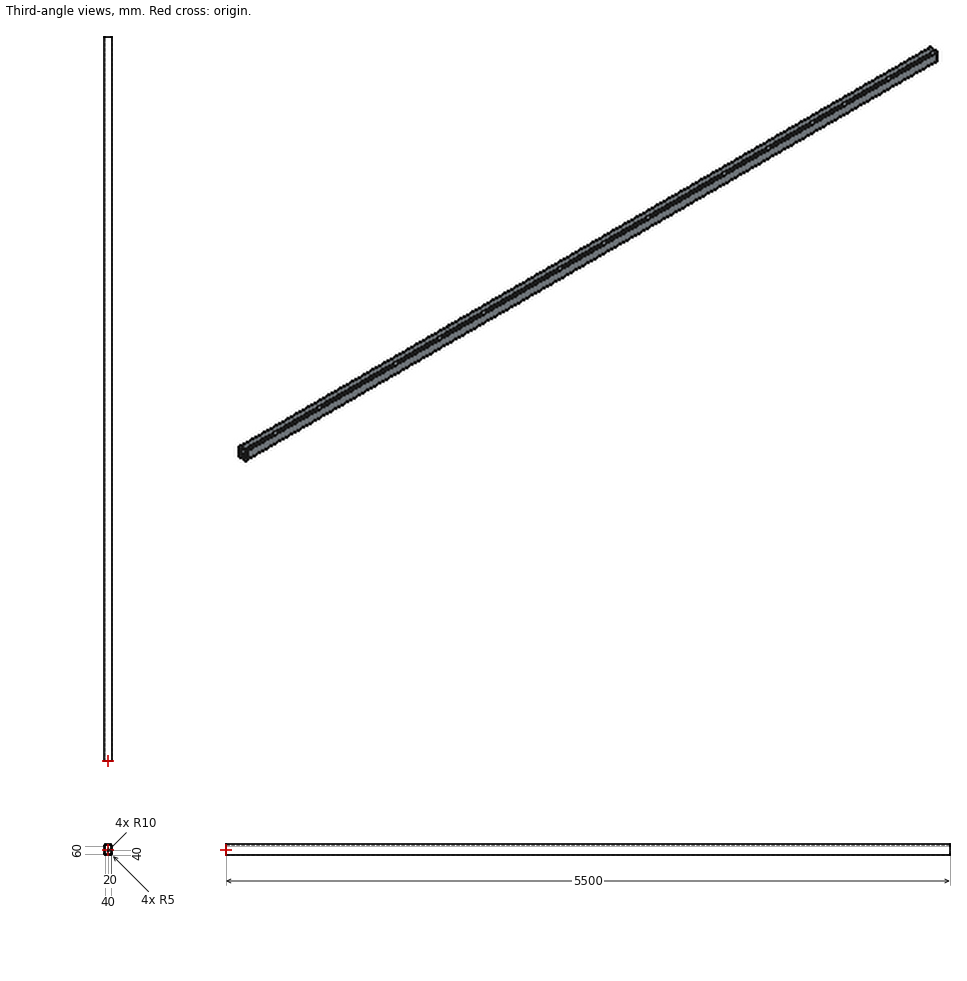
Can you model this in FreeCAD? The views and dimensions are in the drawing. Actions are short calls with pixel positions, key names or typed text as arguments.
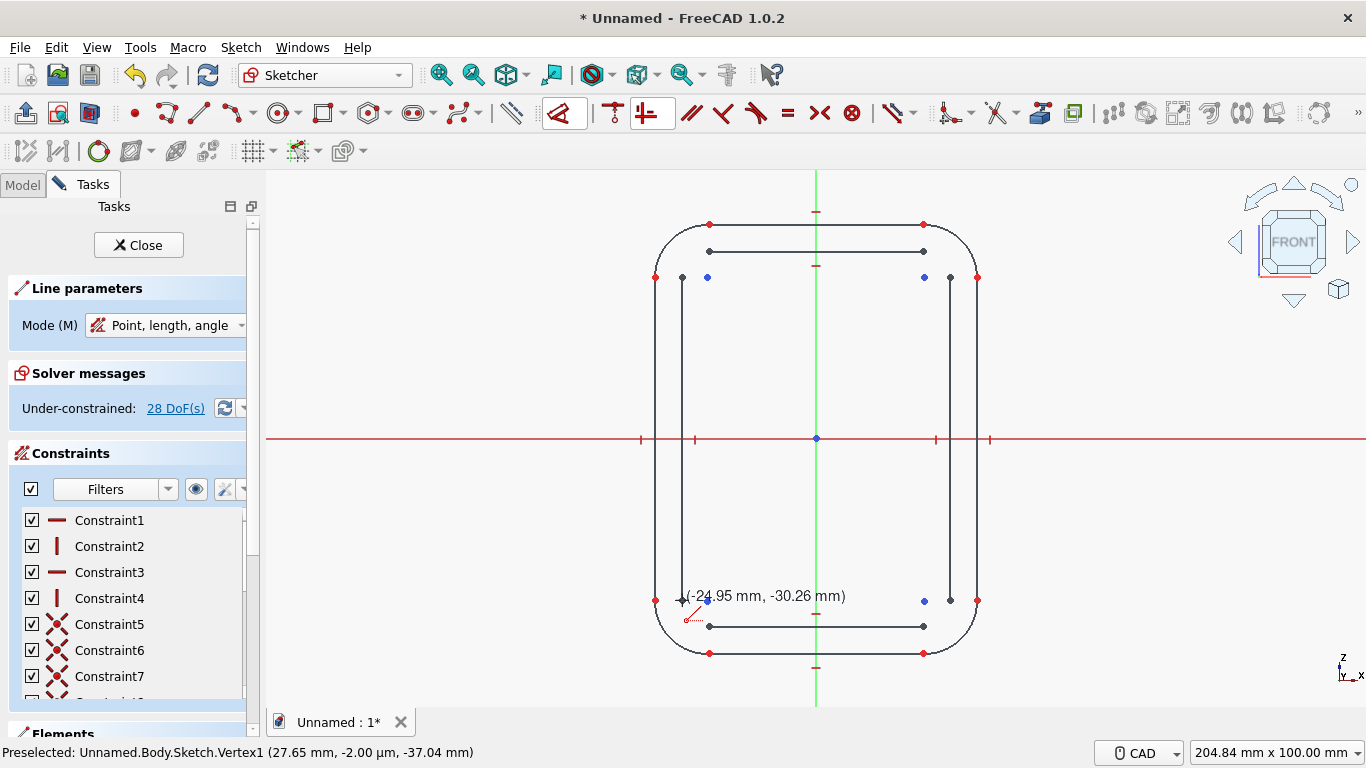
click(232, 114)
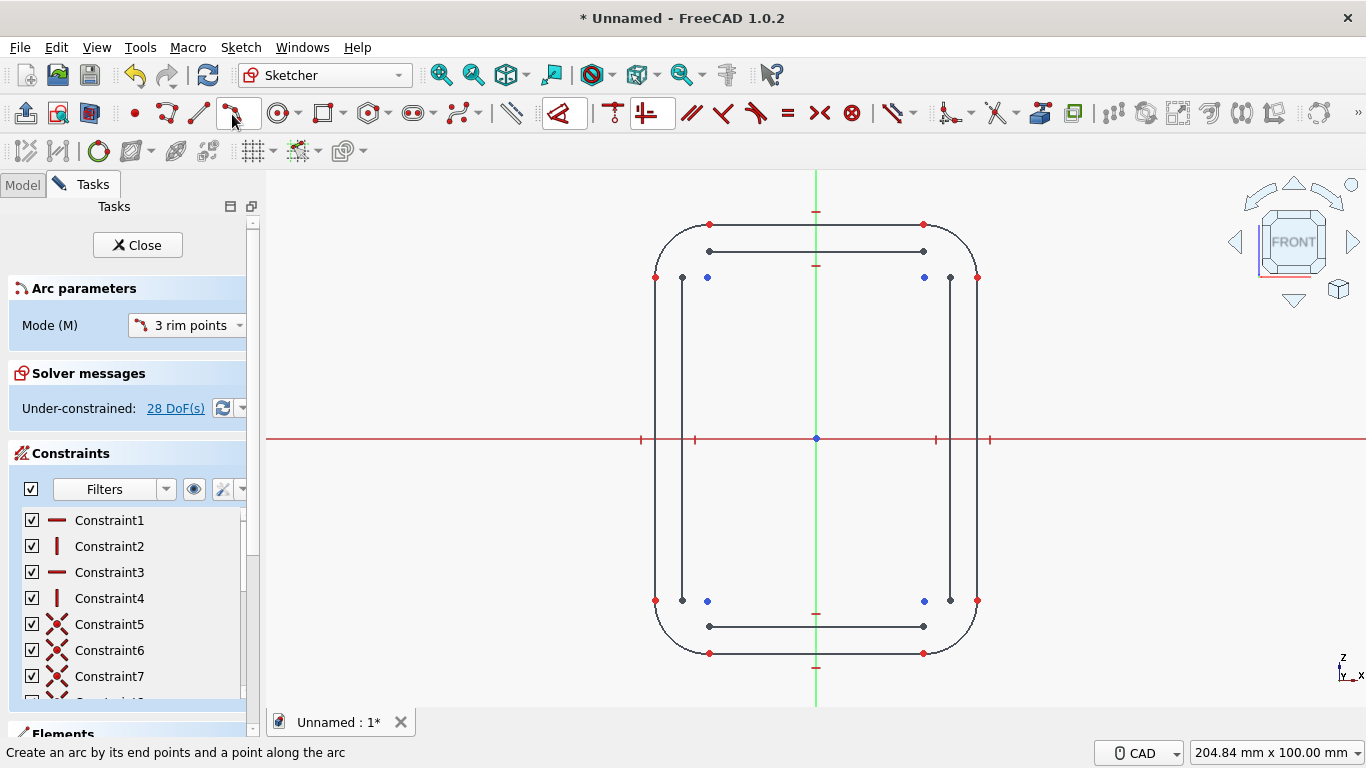
click(923, 627)
click(950, 601)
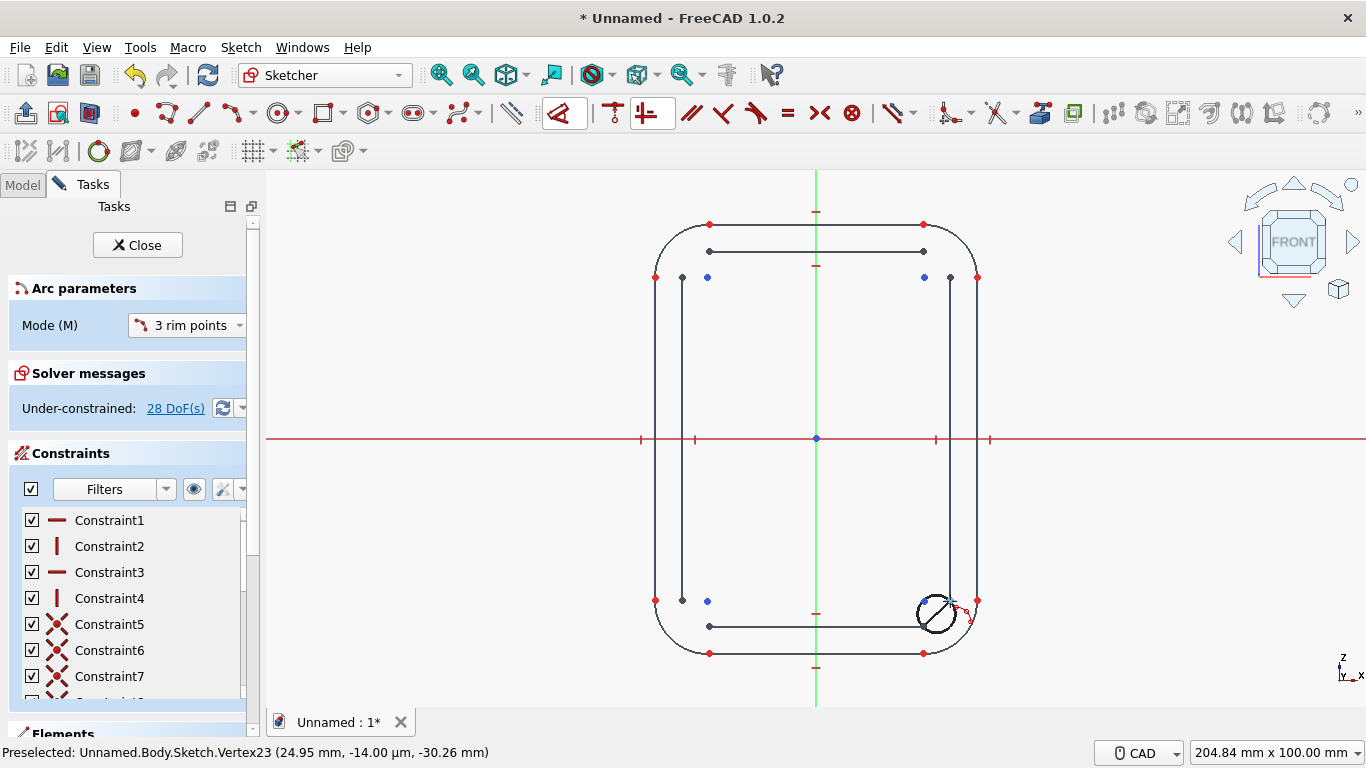
scroll(942, 619, up, 4)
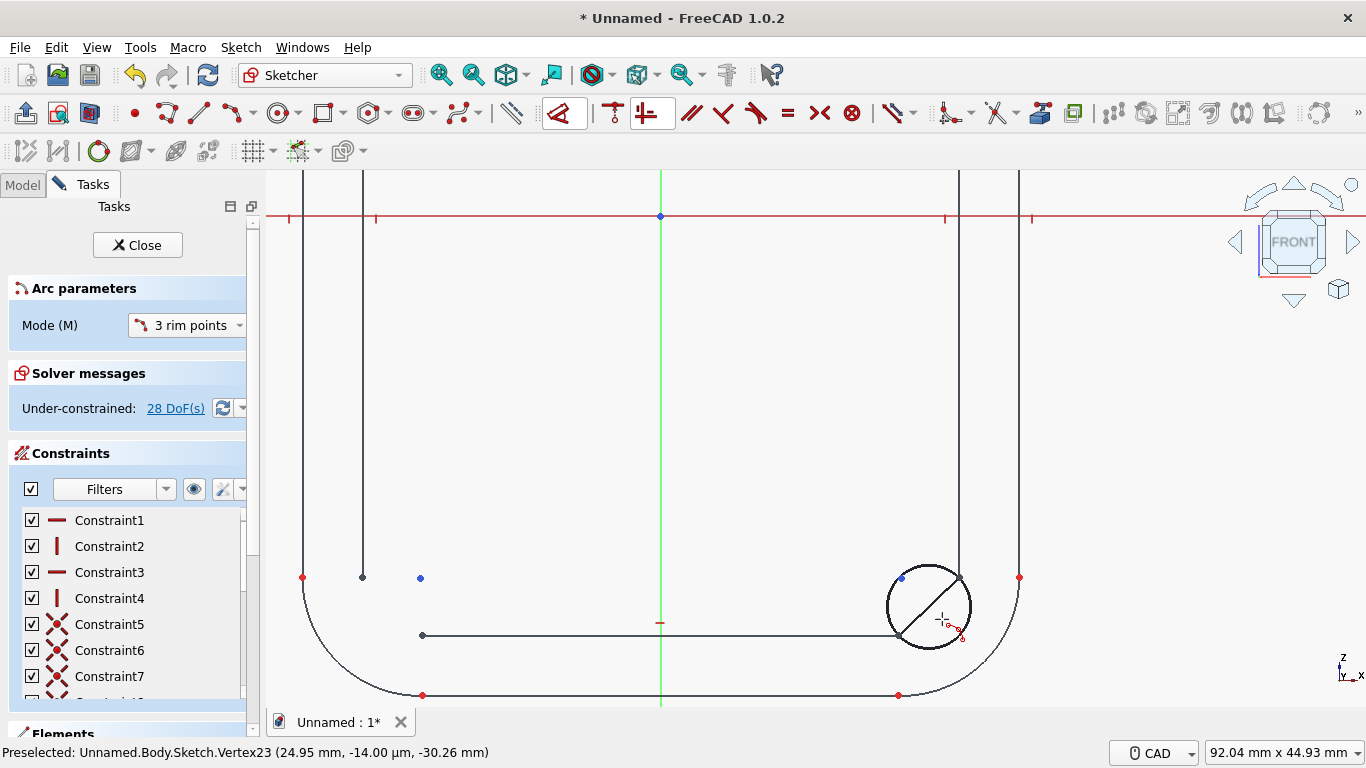
click(942, 617)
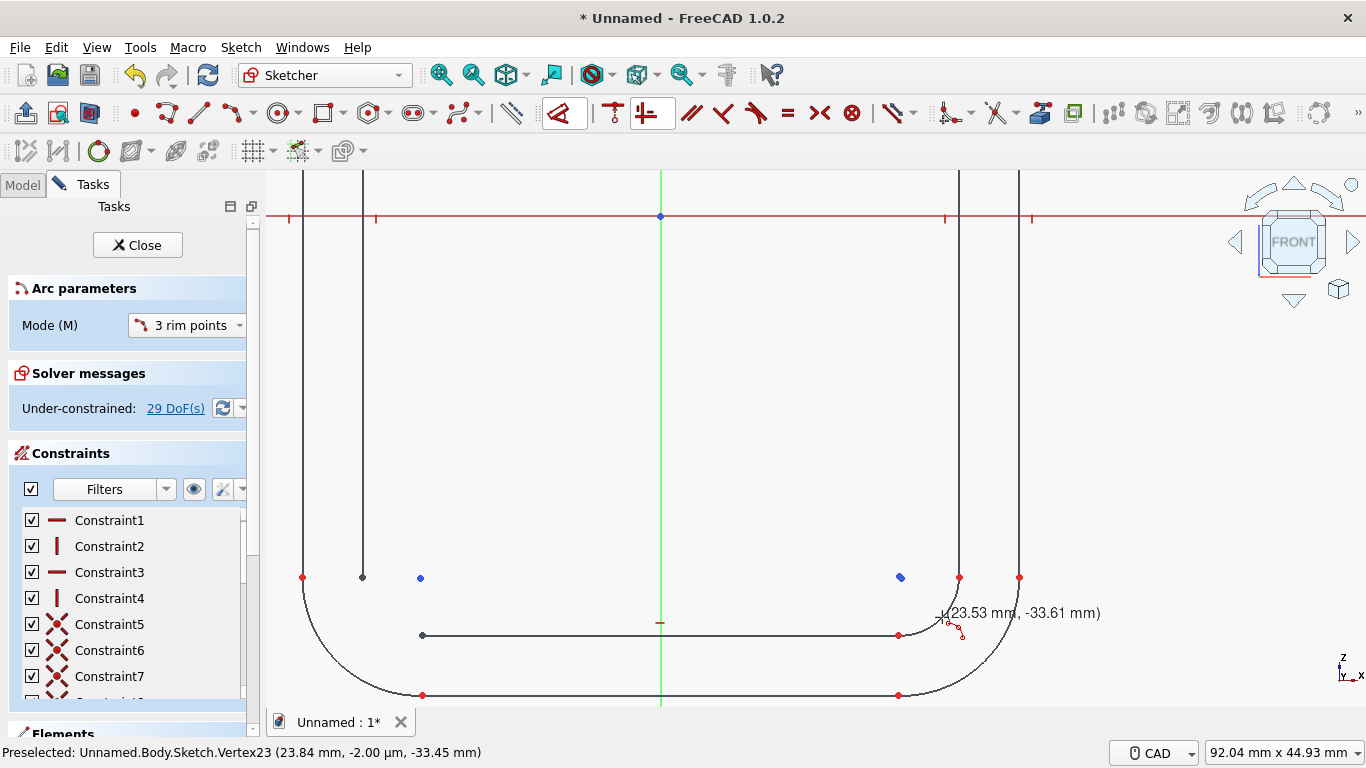
scroll(798, 568, down, 5)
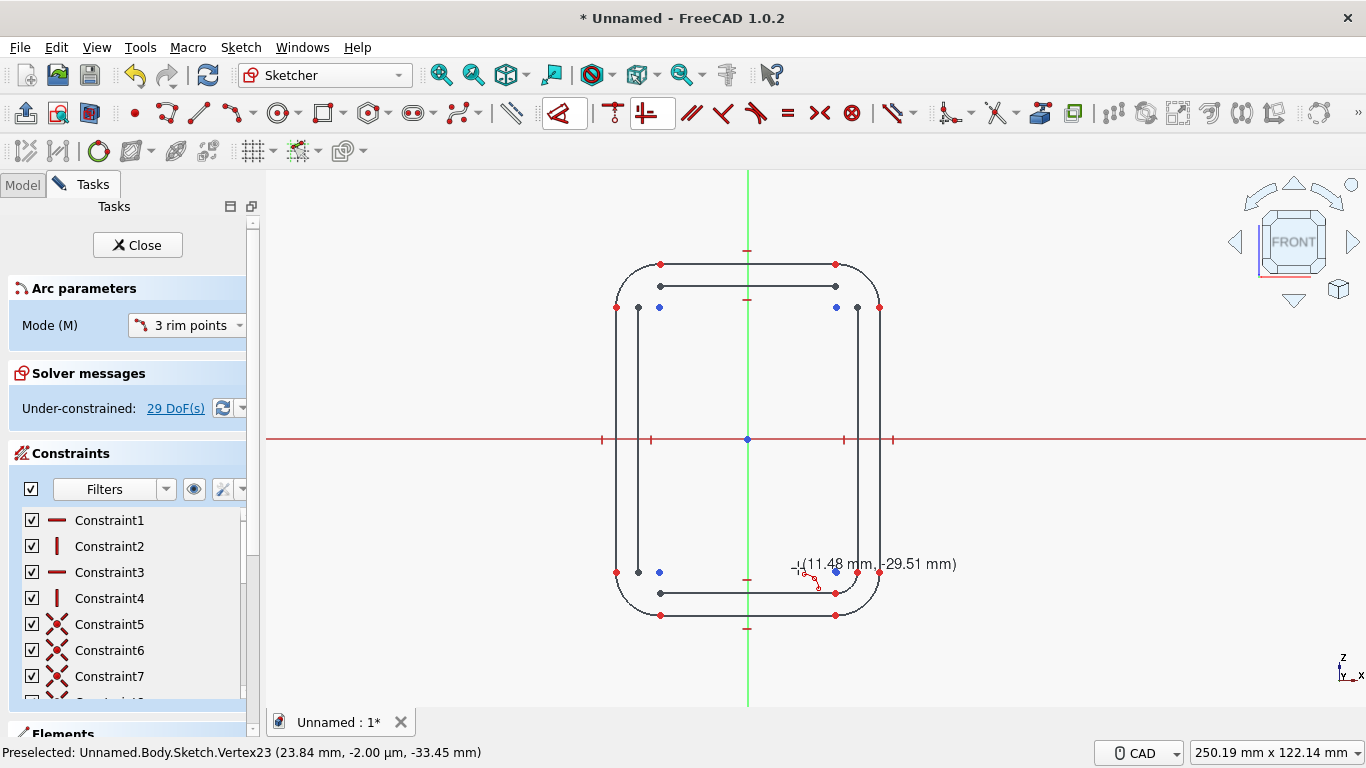
click(858, 308)
click(835, 286)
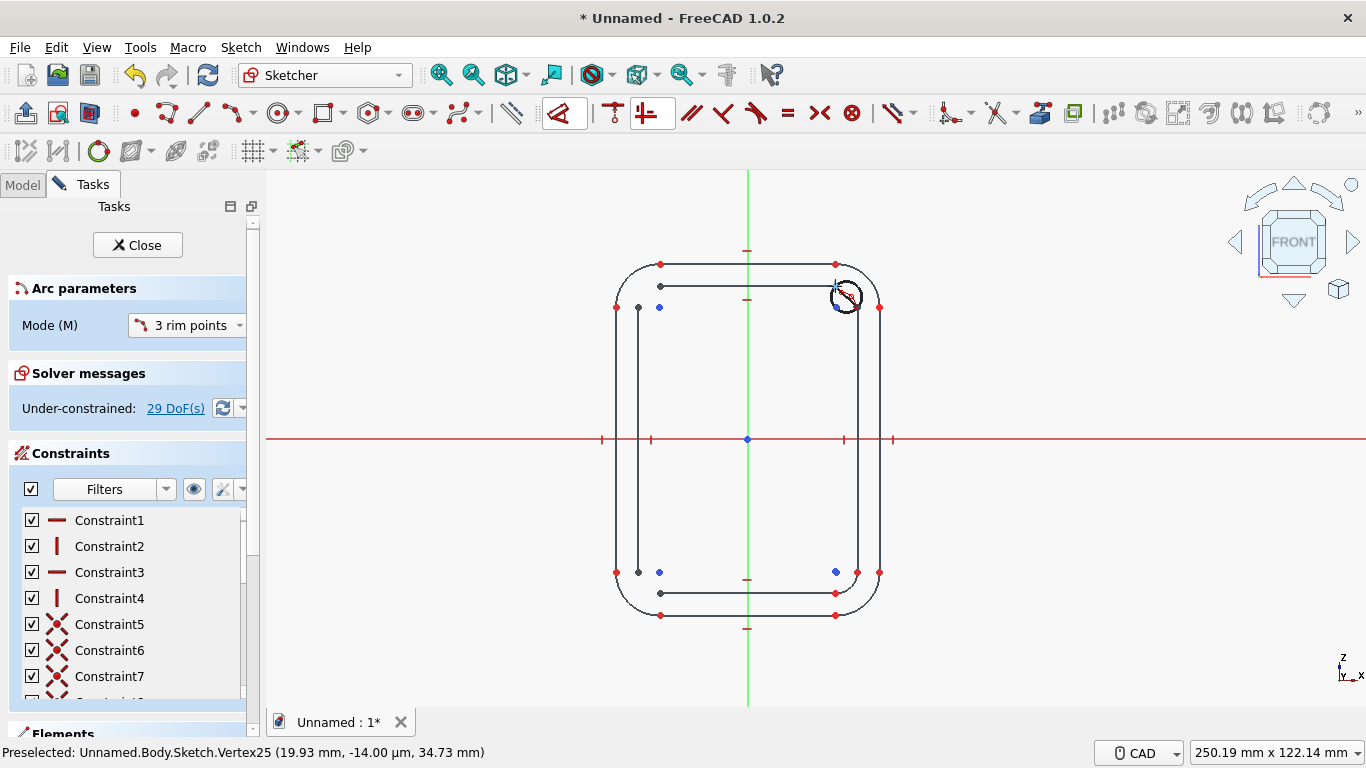
scroll(851, 292, up, 5)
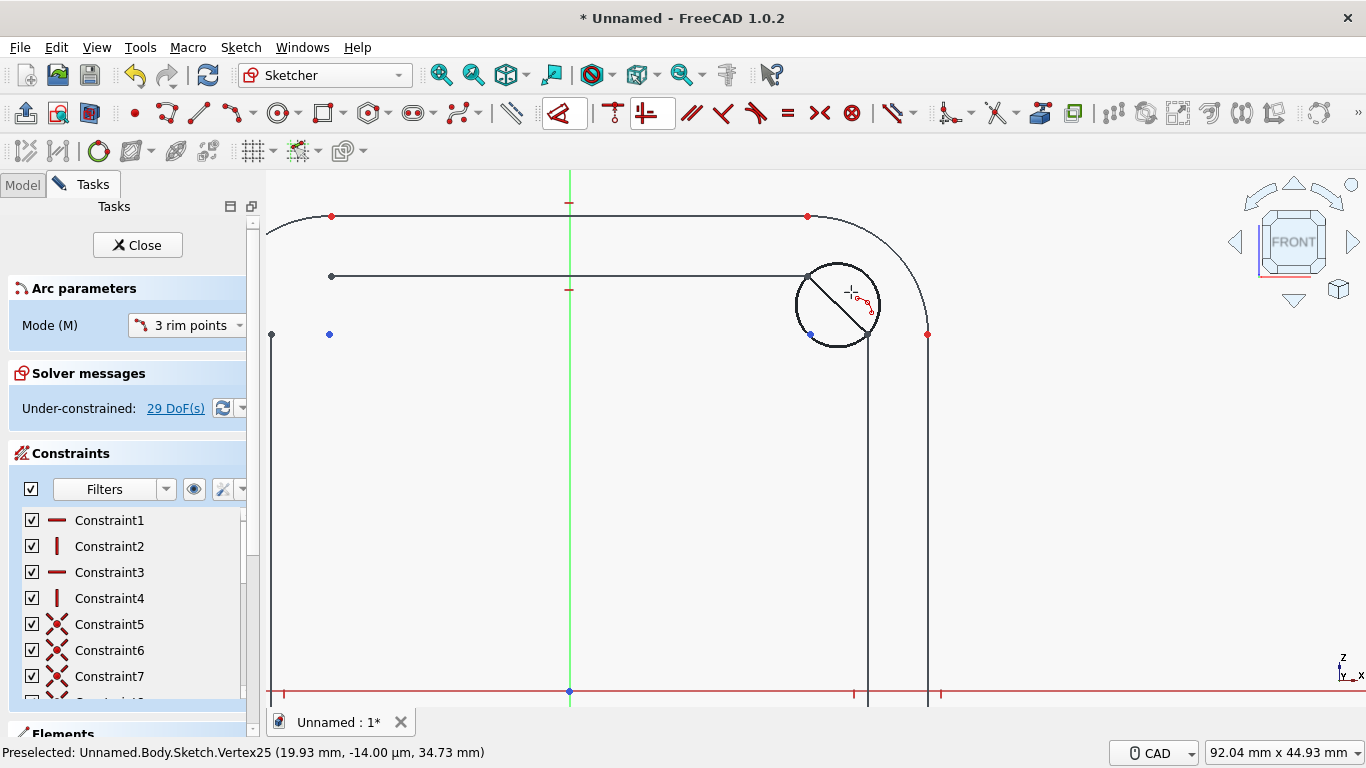
click(851, 291)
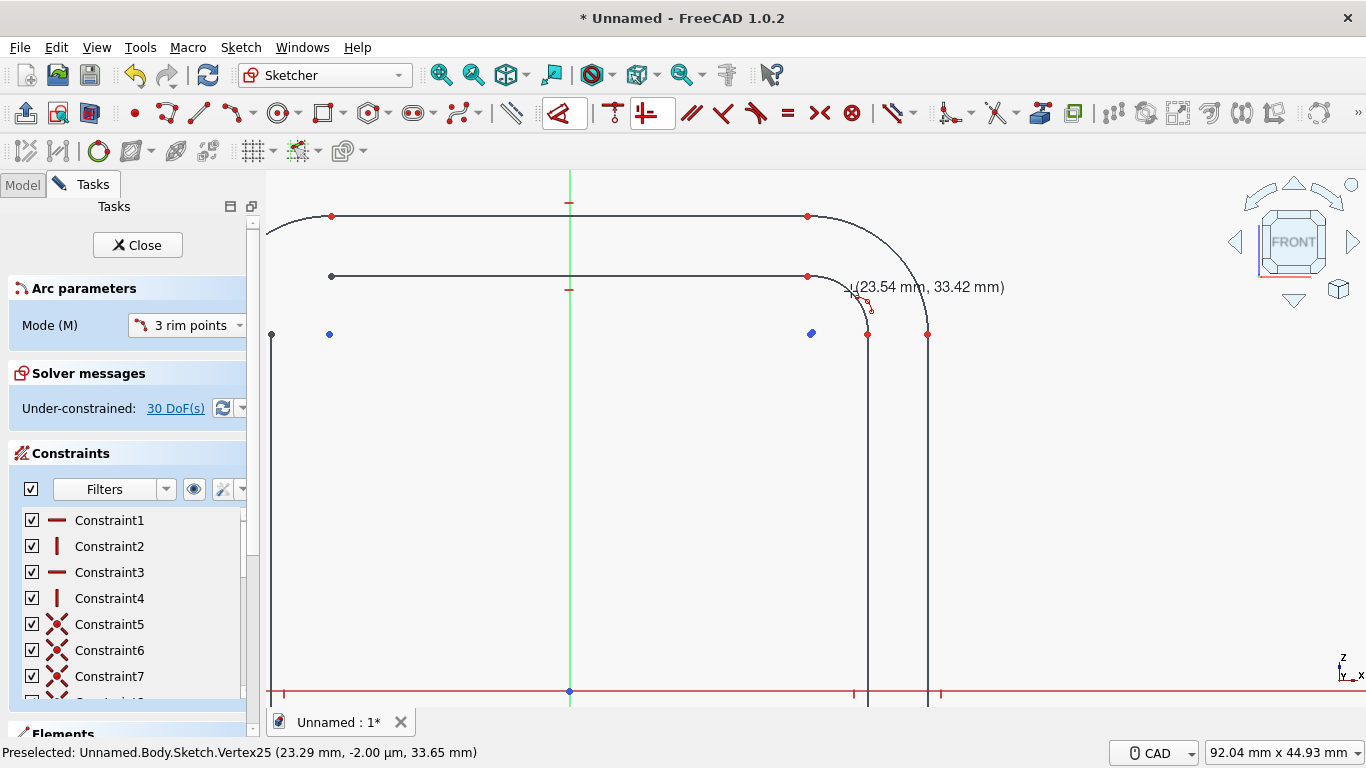
click(332, 276)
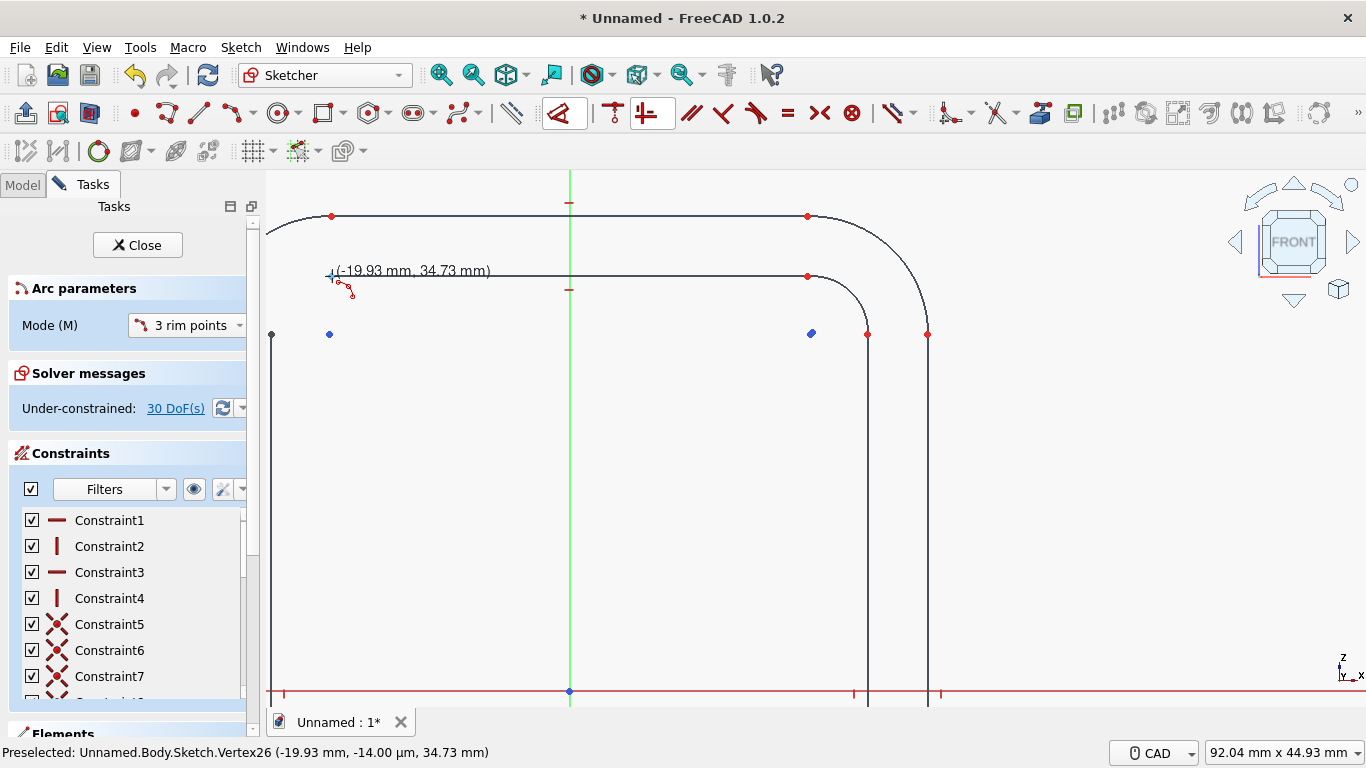
scroll(851, 291, down, 5)